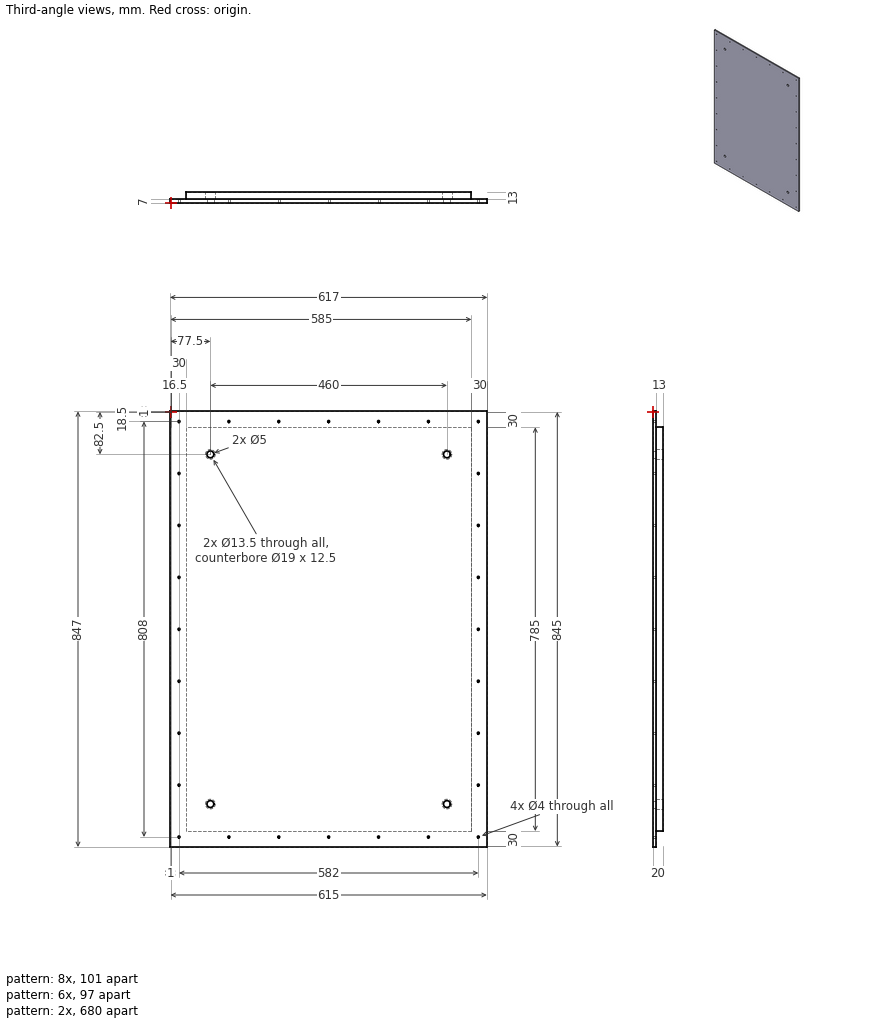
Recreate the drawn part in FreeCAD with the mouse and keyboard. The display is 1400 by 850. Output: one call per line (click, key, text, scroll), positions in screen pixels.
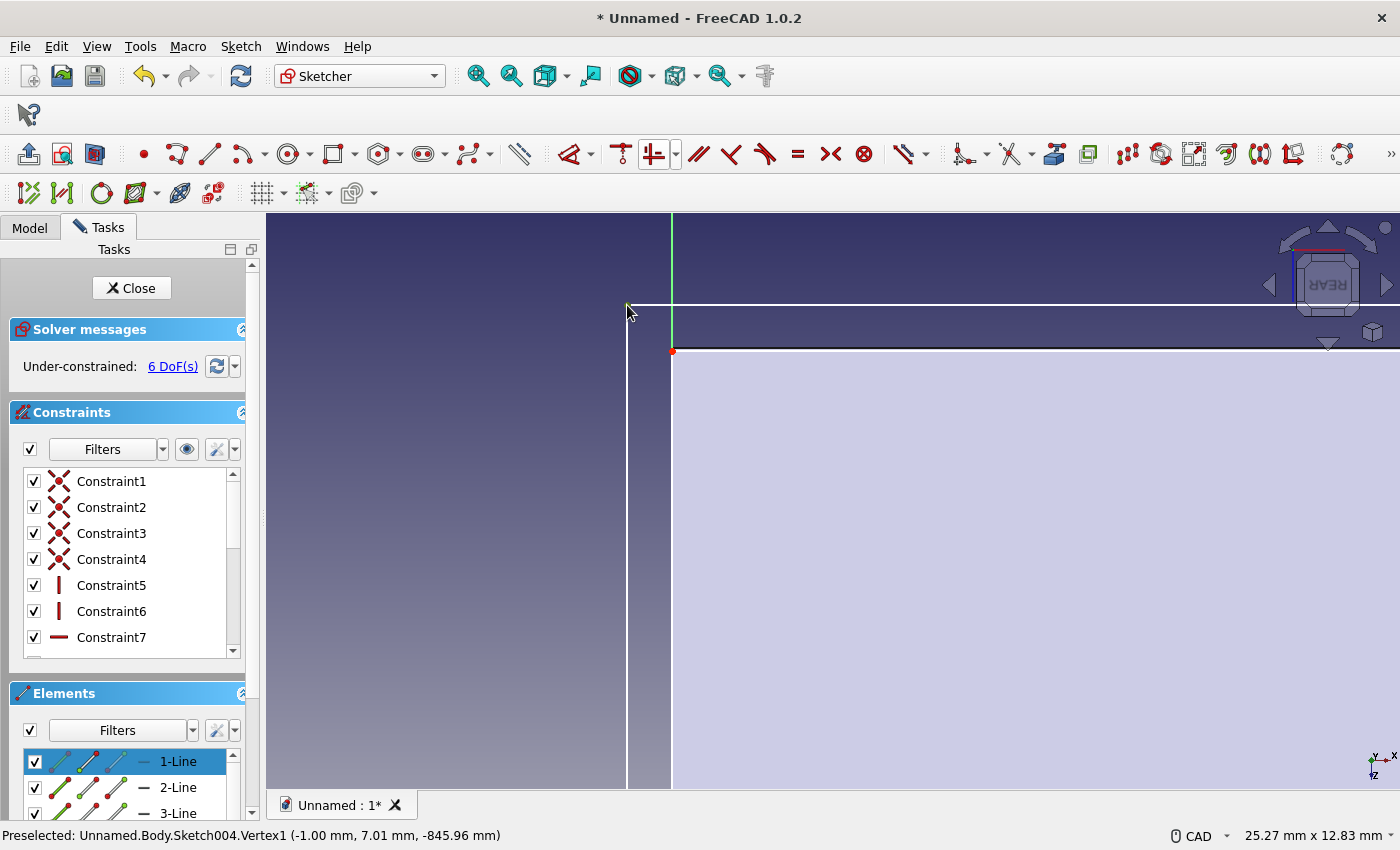
key(l)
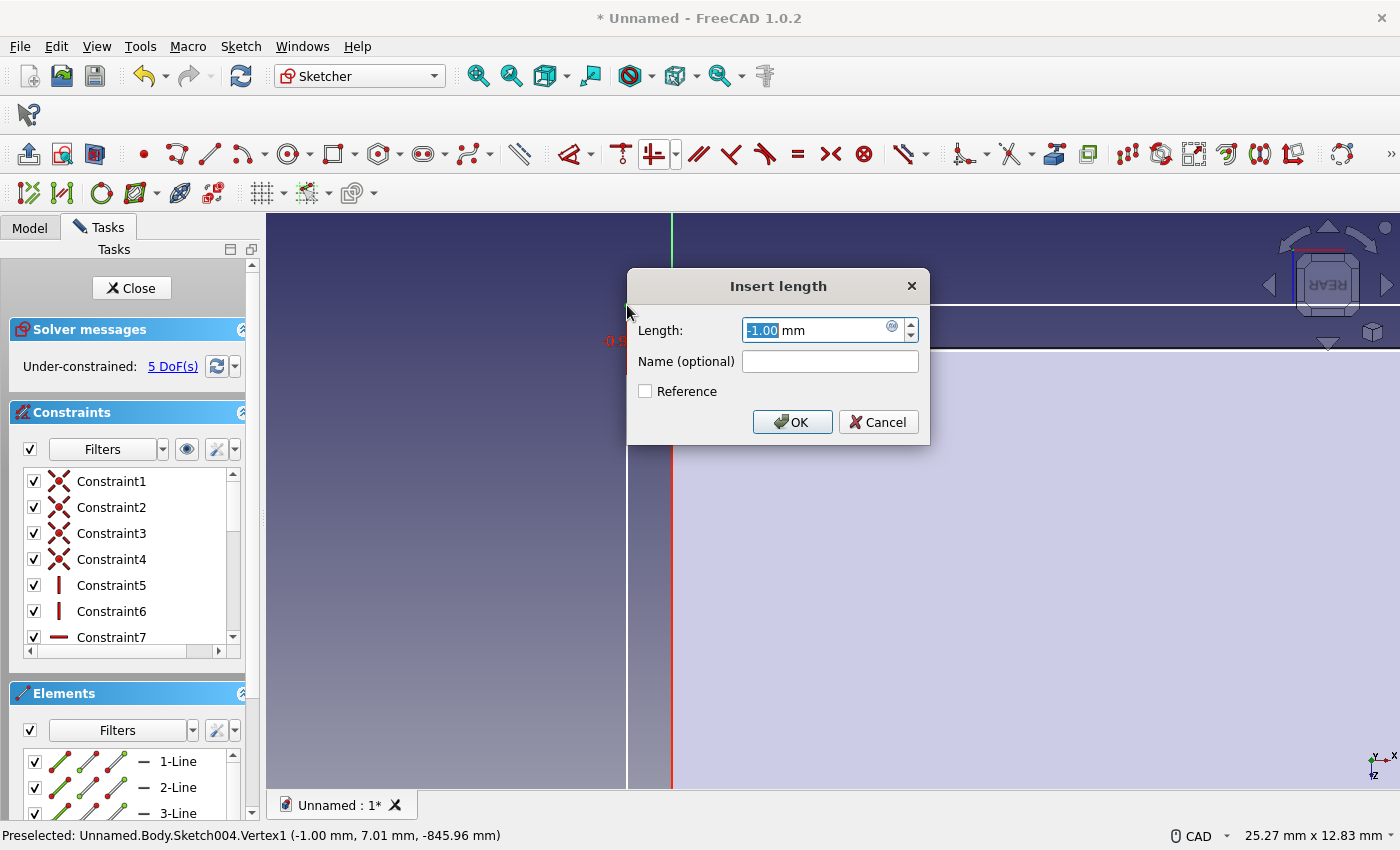
text(-1)
key(Return)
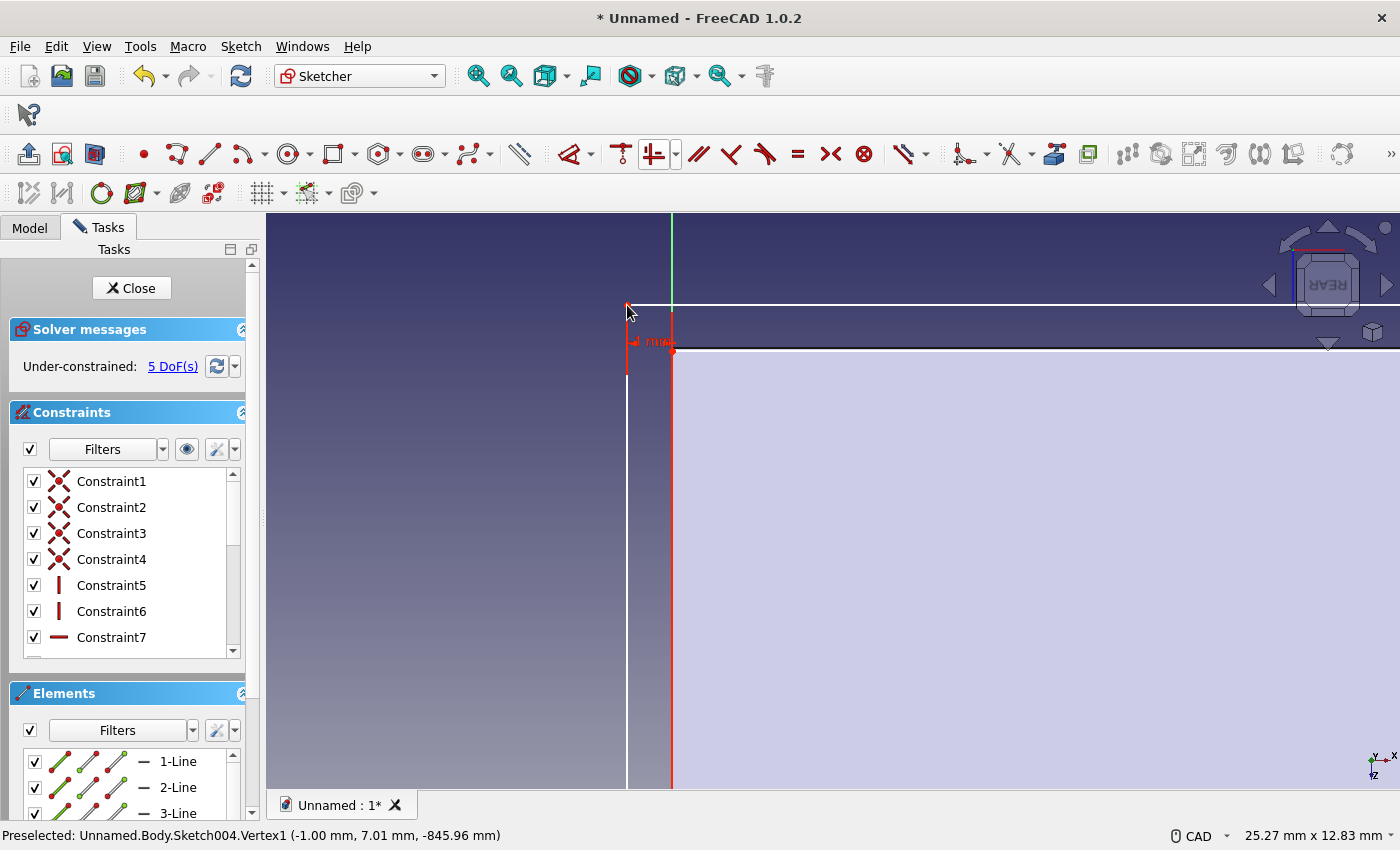
scroll(764, 501, down, 15)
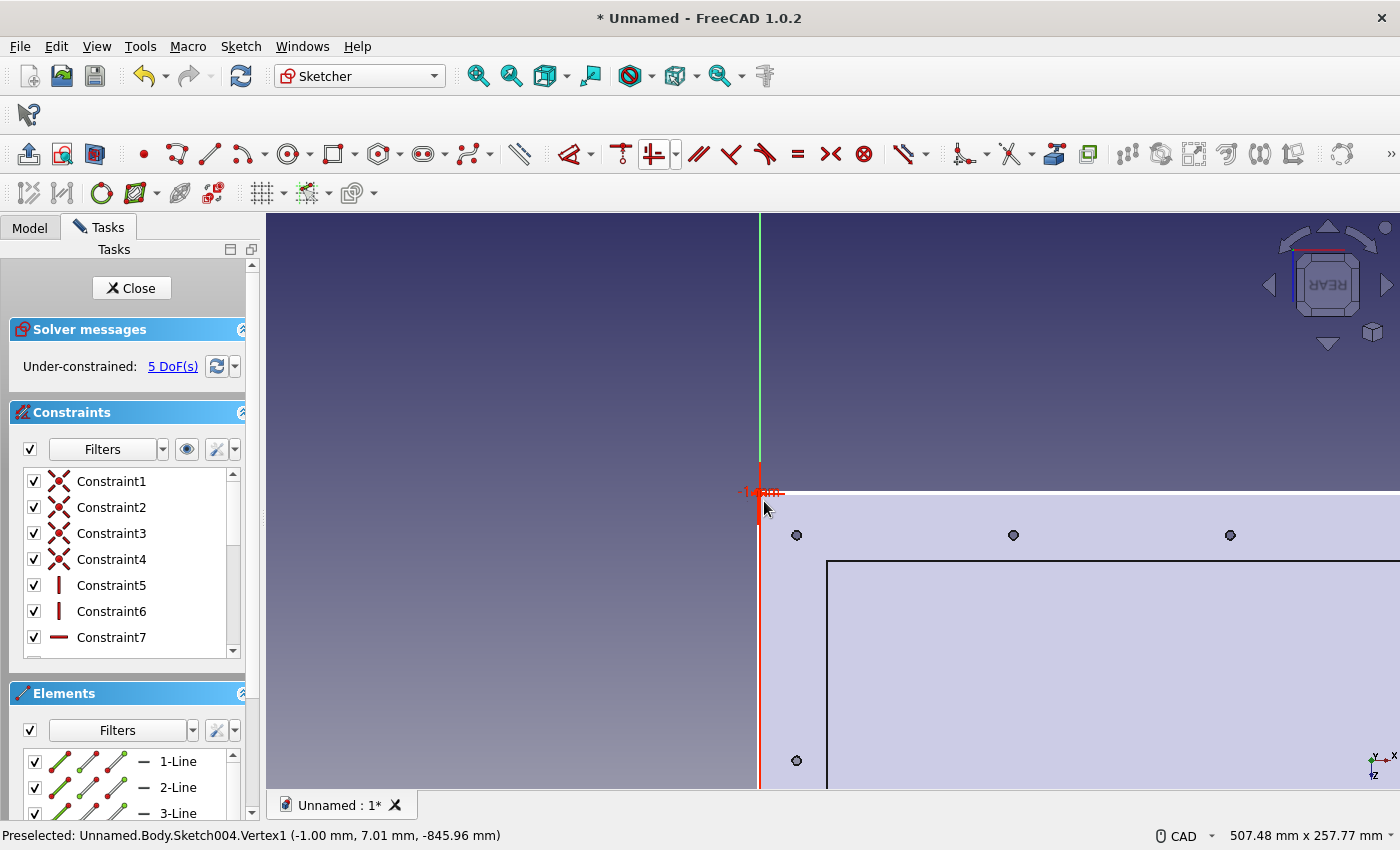
scroll(592, 264, down, 8)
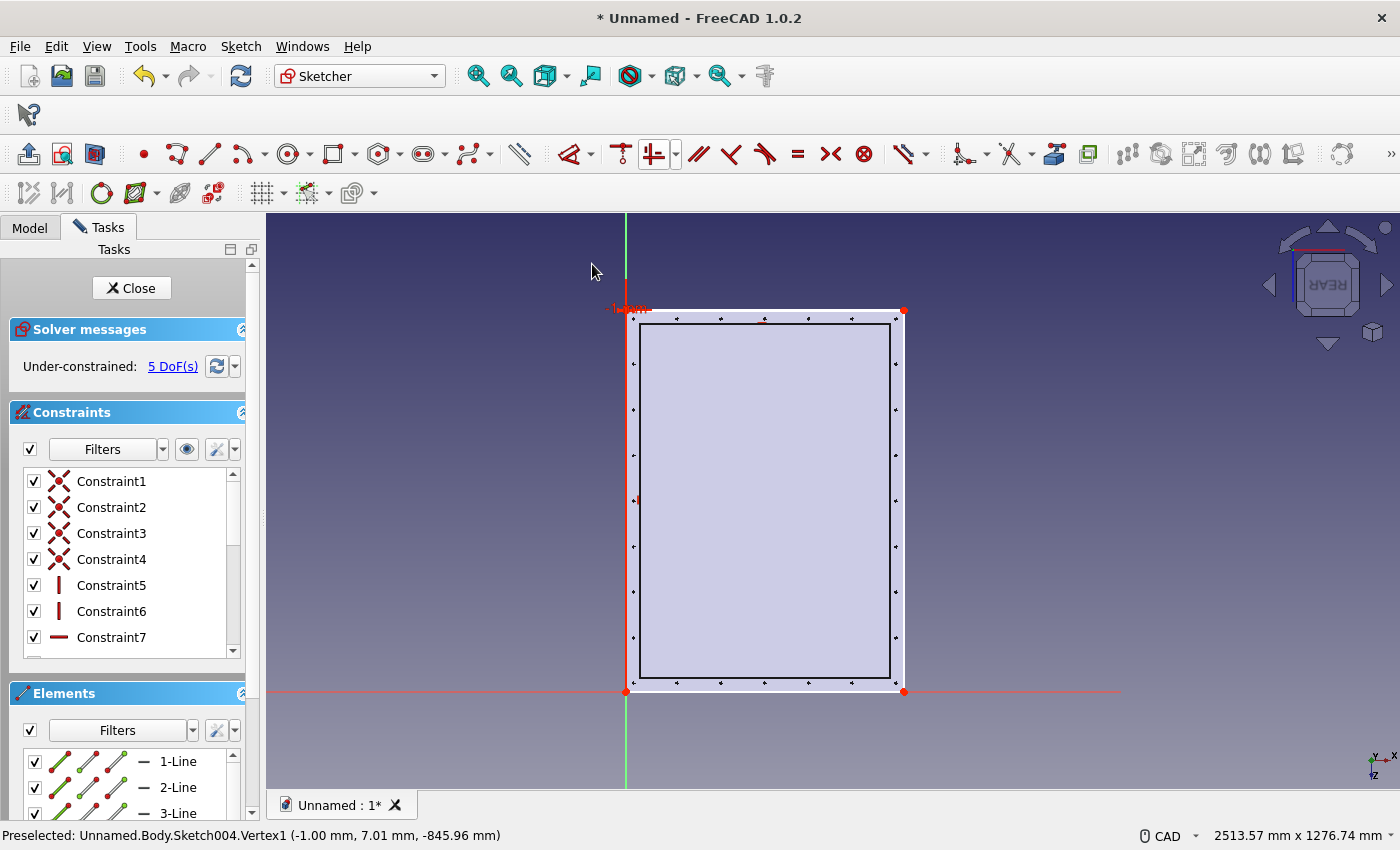
scroll(626, 692, up, 23)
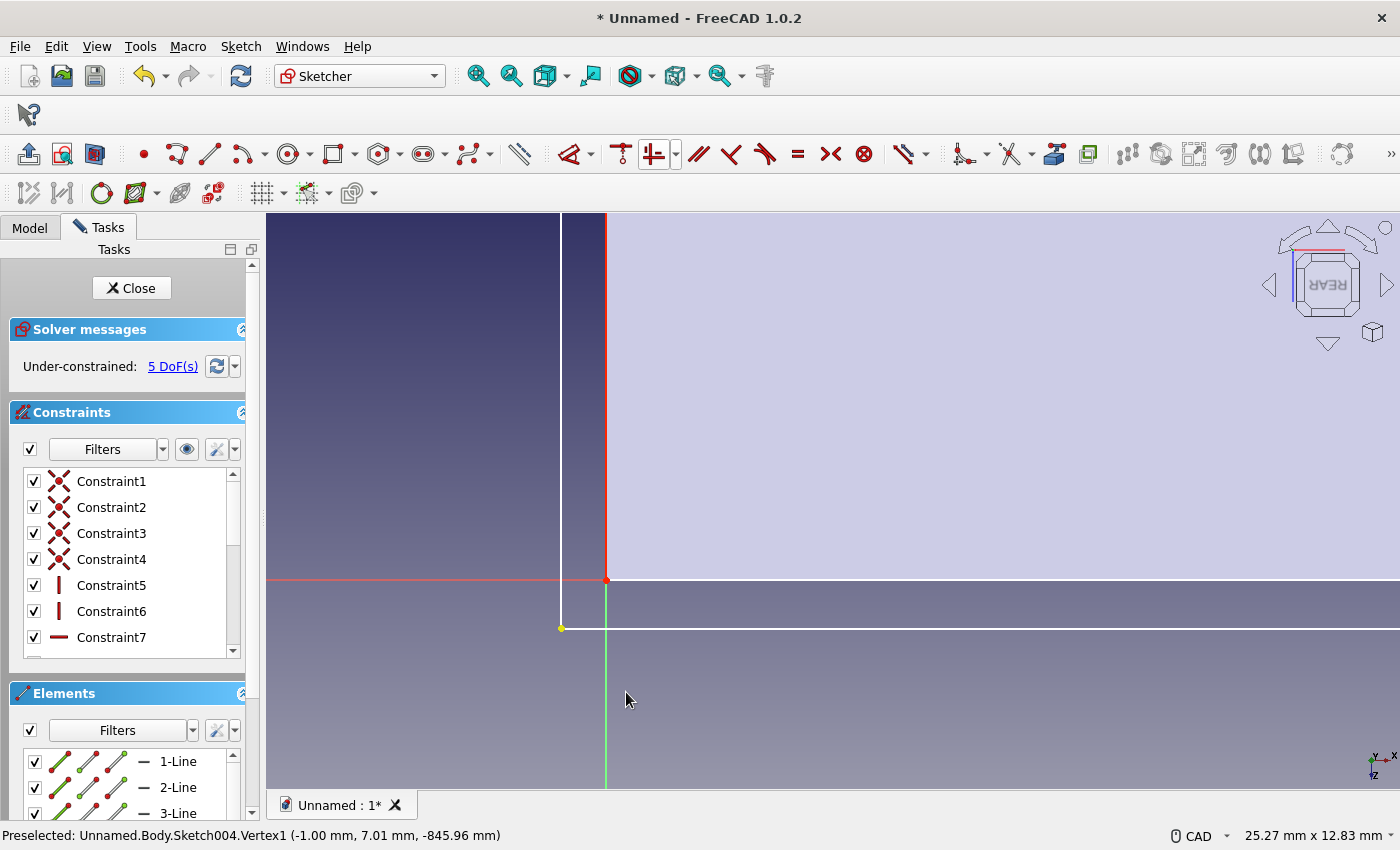
click(562, 629)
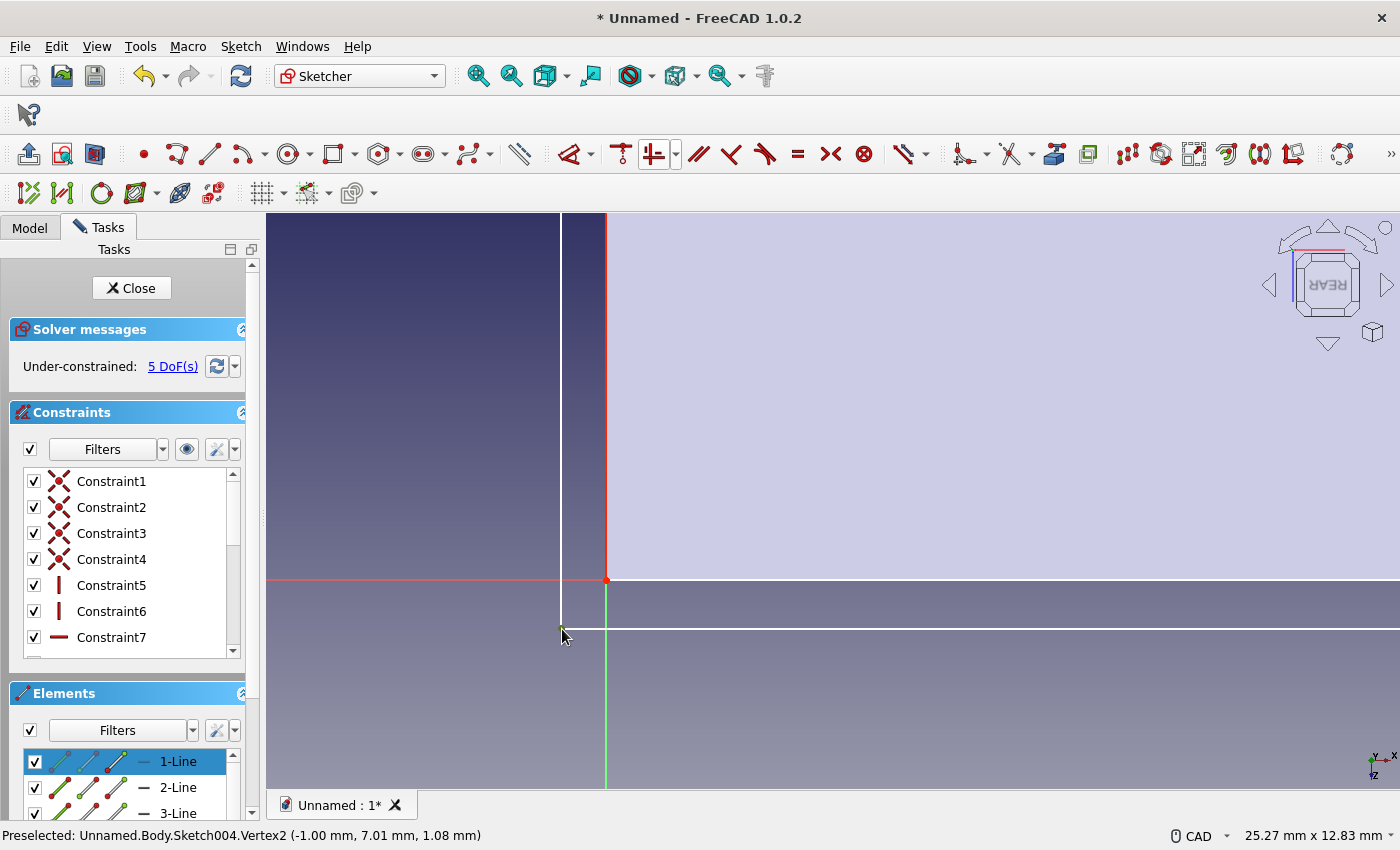
key(i)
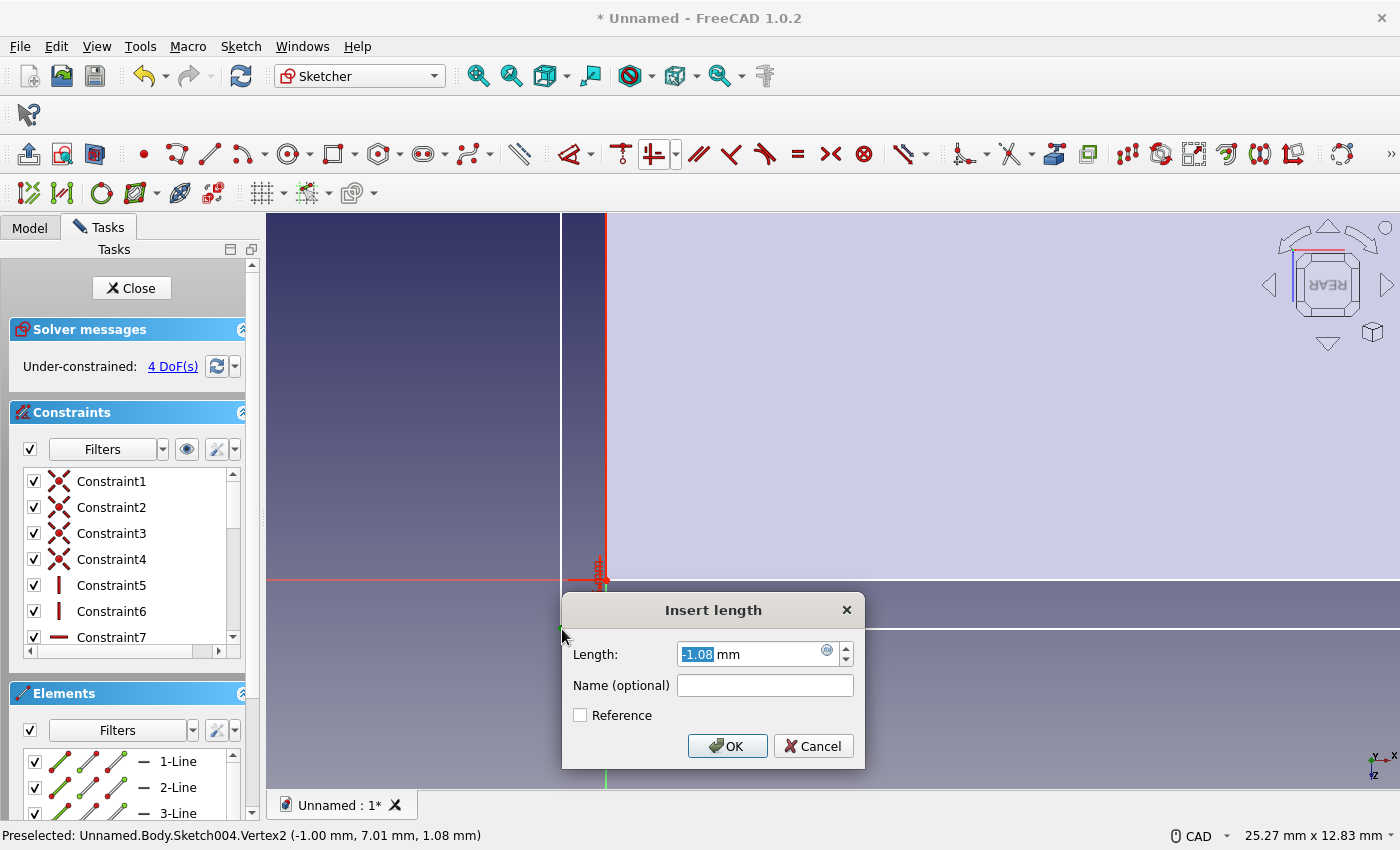
text(-1)
key(Return)